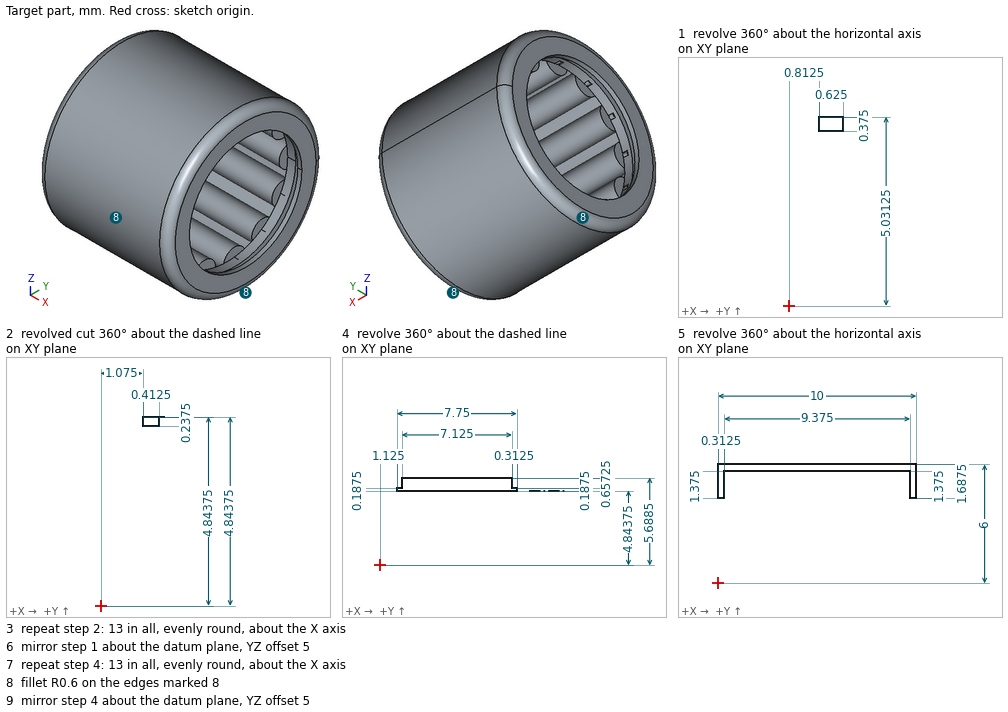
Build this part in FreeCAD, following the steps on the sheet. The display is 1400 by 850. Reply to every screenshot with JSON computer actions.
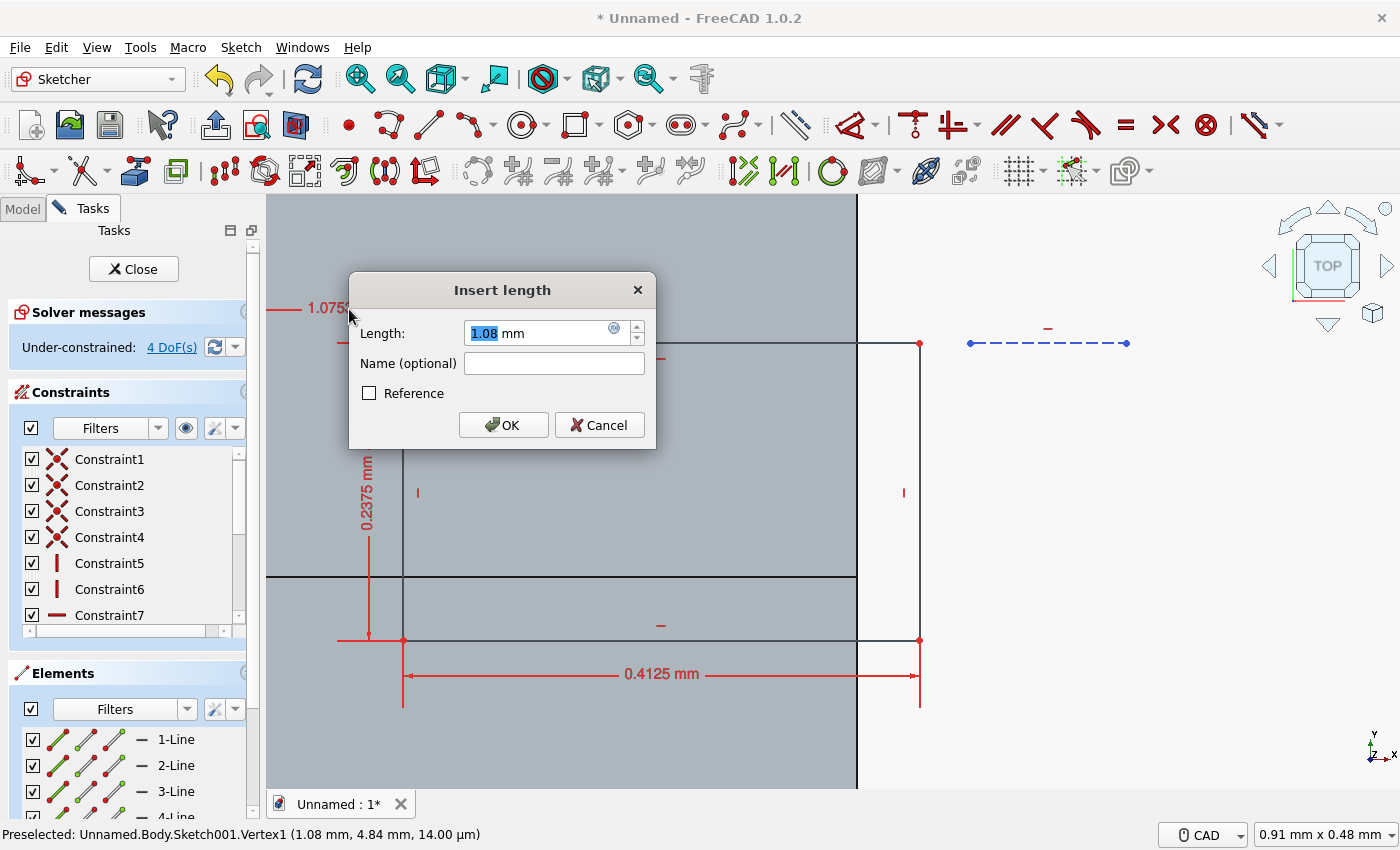
{"action": "type", "text": "1.075"}
{"action": "key", "text": "Return"}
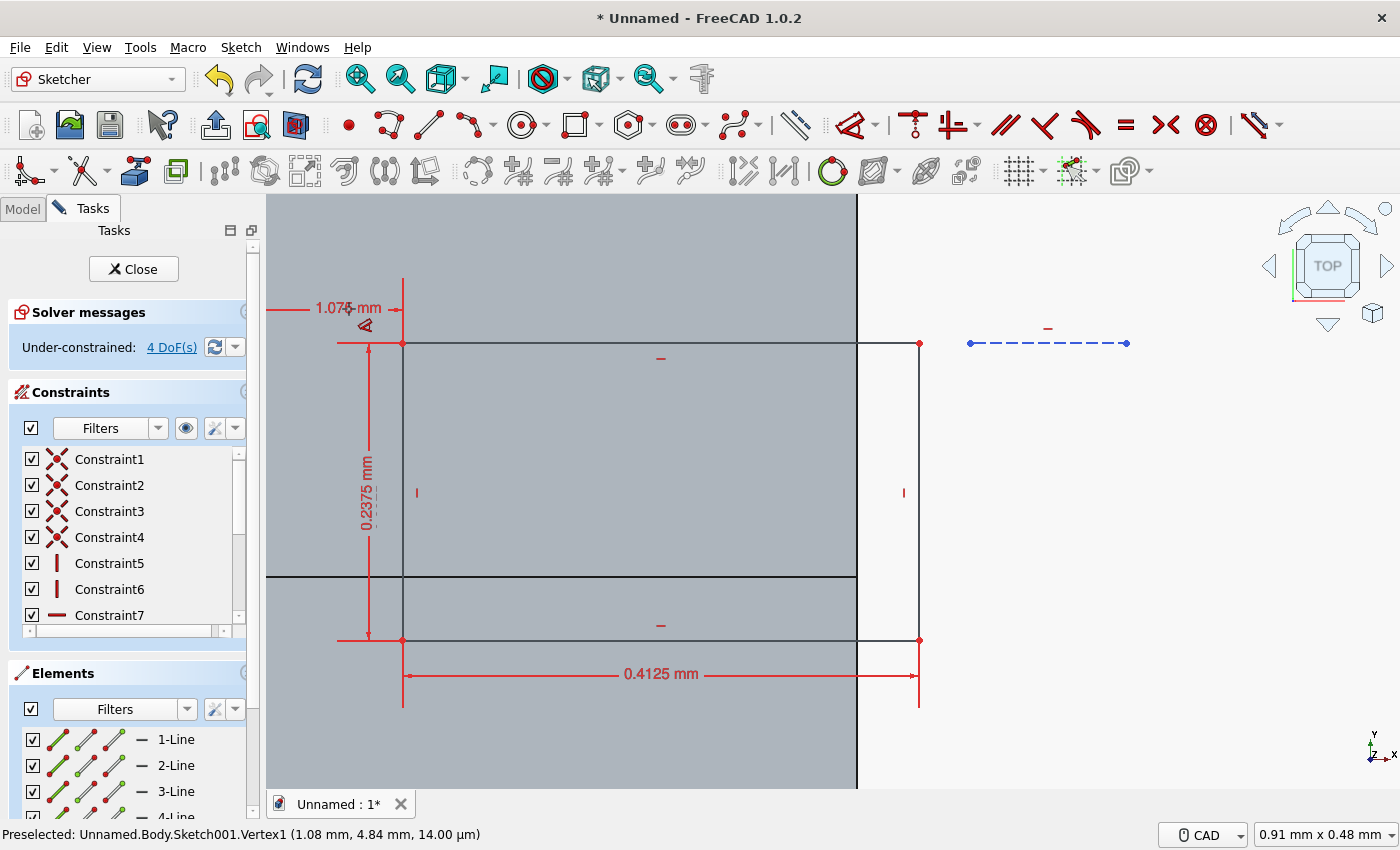
{"action": "left_click", "coordinate": [403, 343]}
{"action": "left_click", "coordinate": [437, 552]}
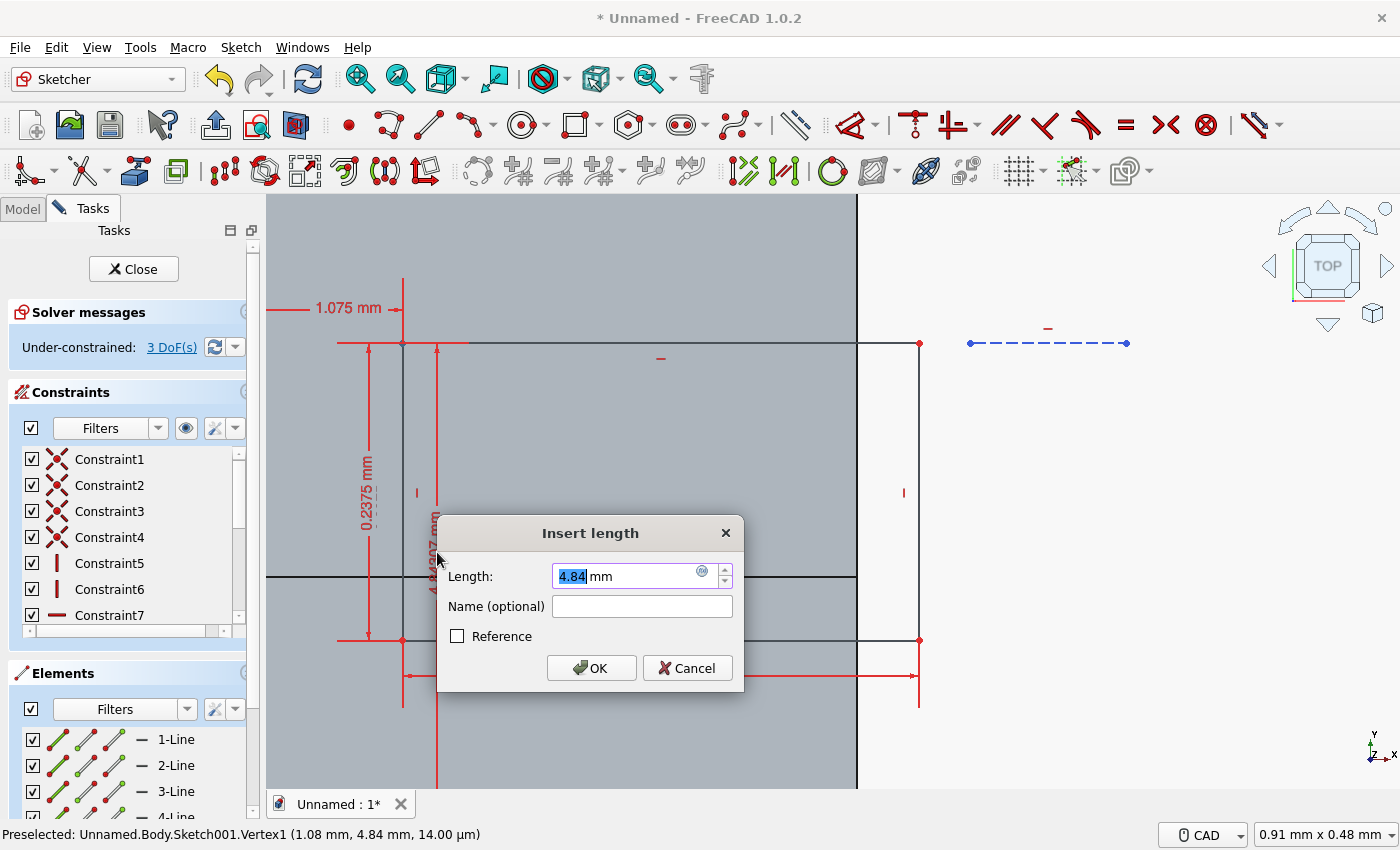
{"action": "type", "text": "4.84375"}
{"action": "key", "text": "Return"}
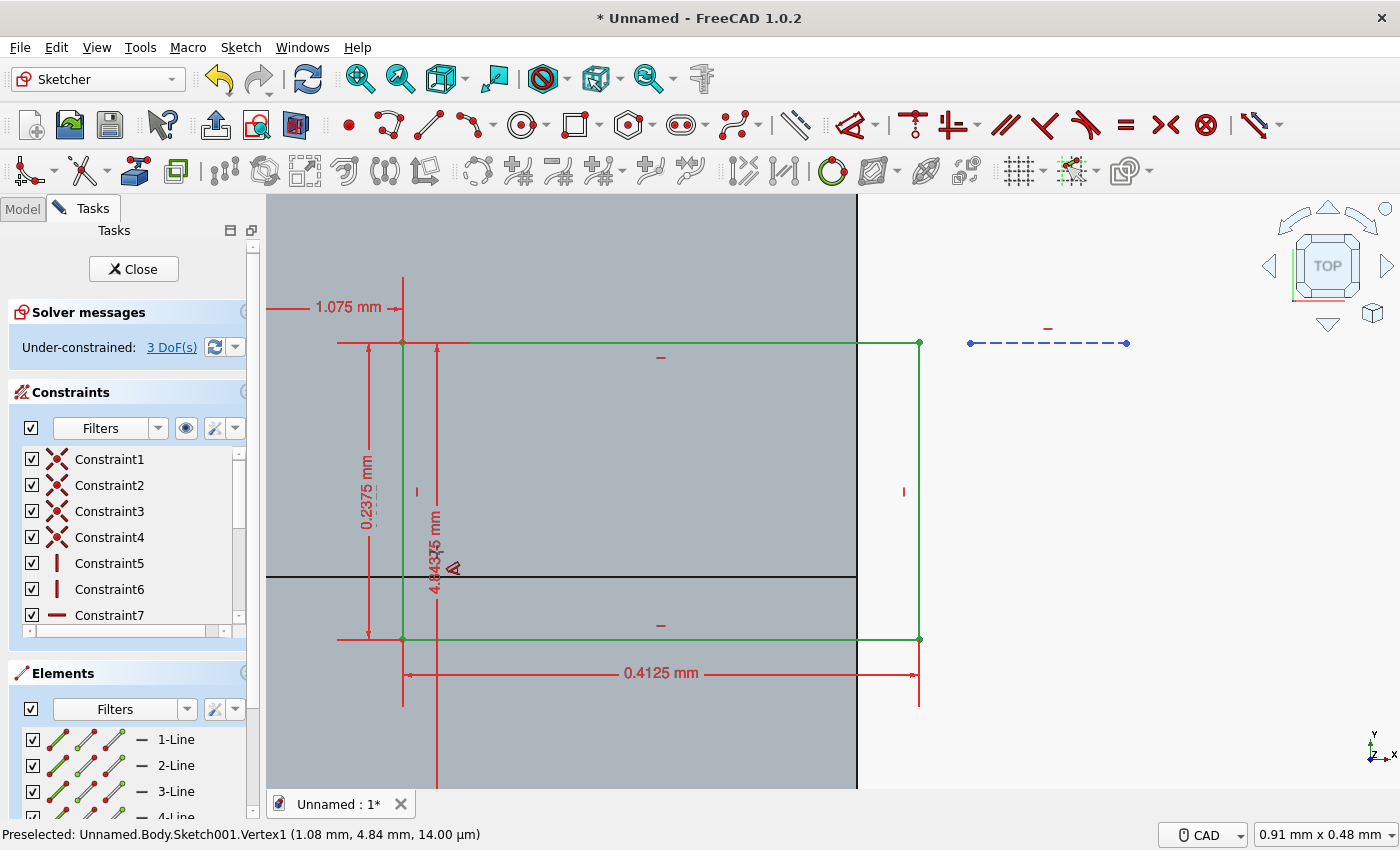
{"action": "left_click", "coordinate": [971, 343]}
{"action": "left_click", "coordinate": [1005, 552]}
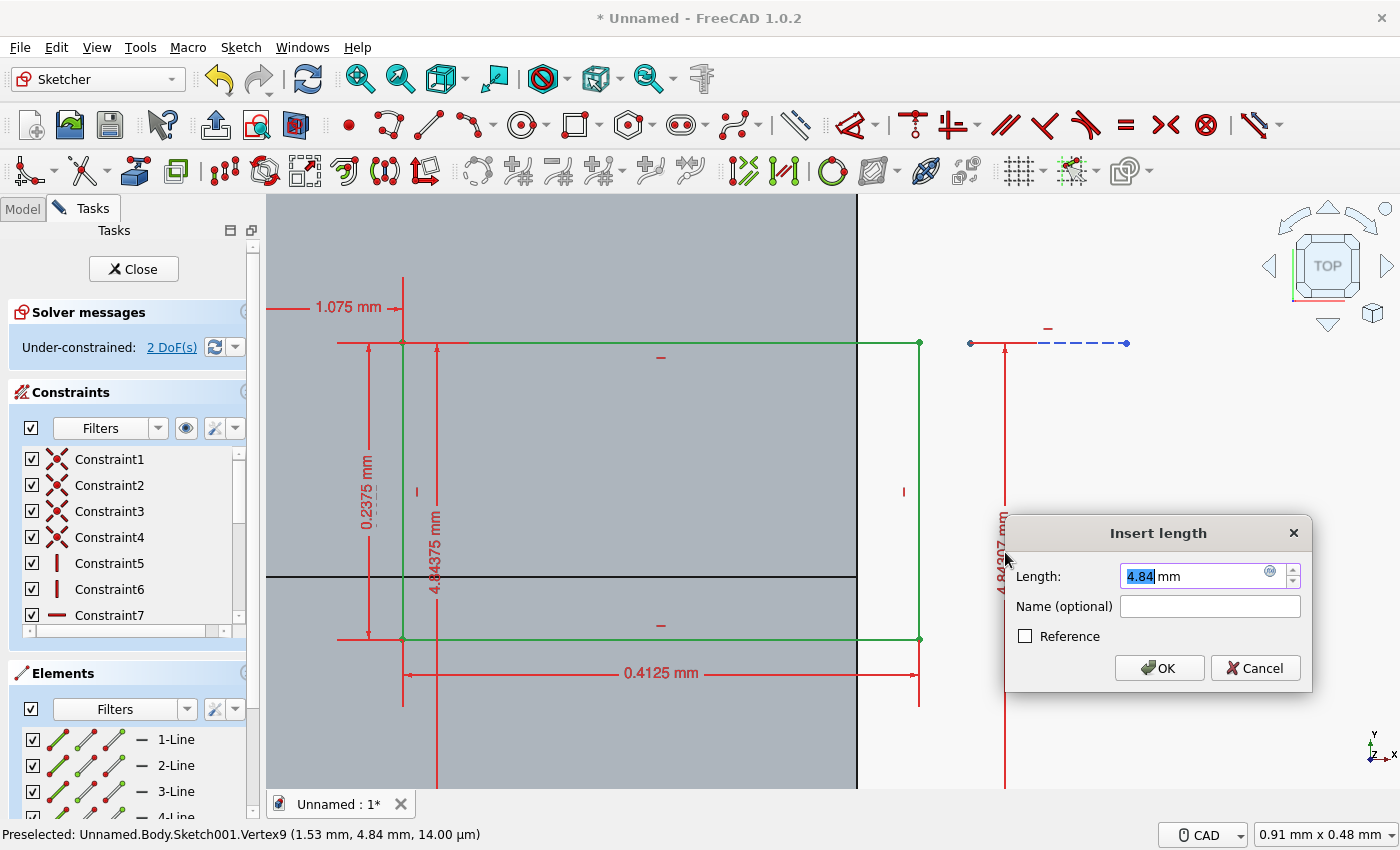
{"action": "type", "text": "4.84375"}
{"action": "key", "text": "Return"}
{"action": "key", "text": "Escape"}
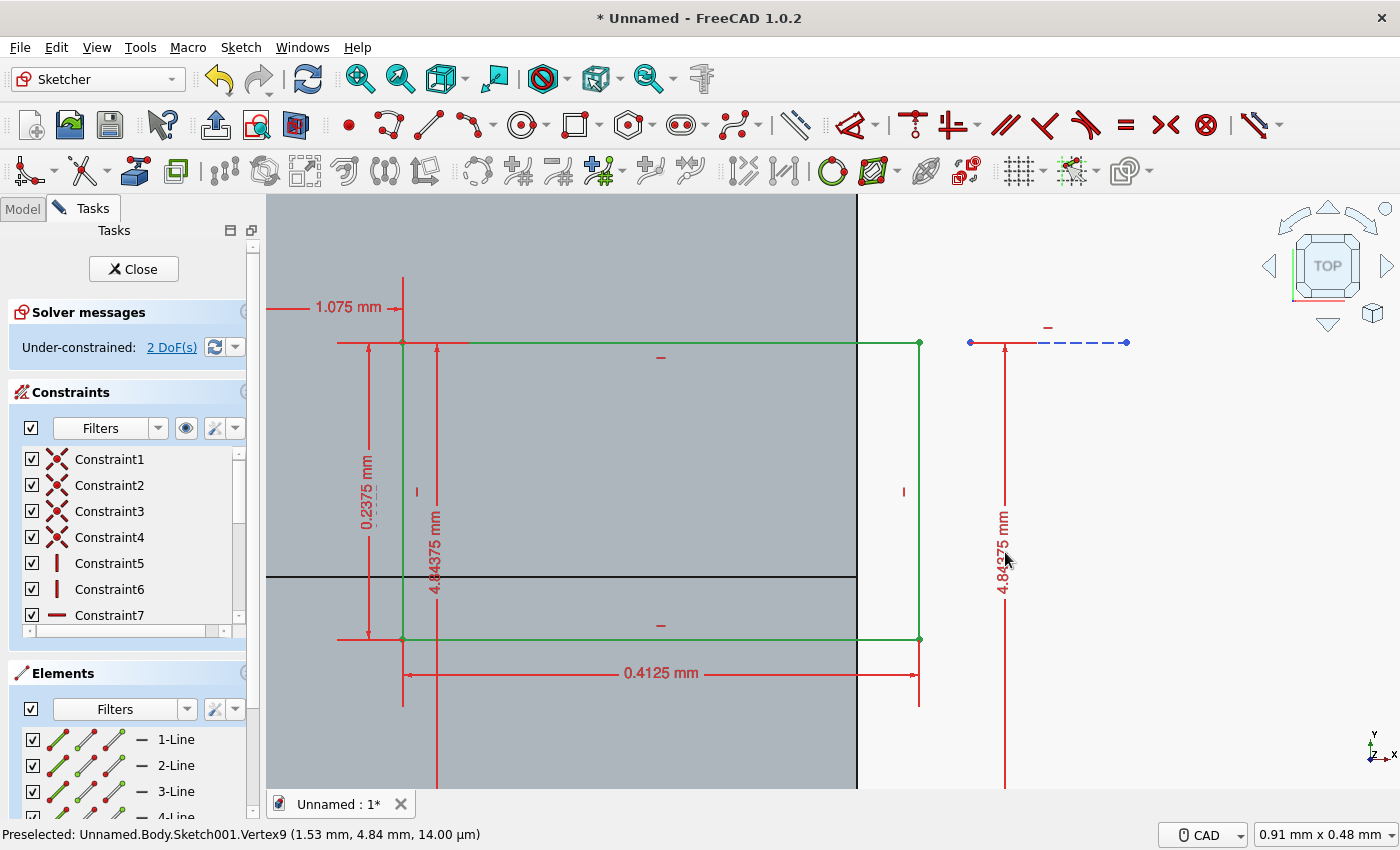
{"action": "left_click", "coordinate": [134, 269]}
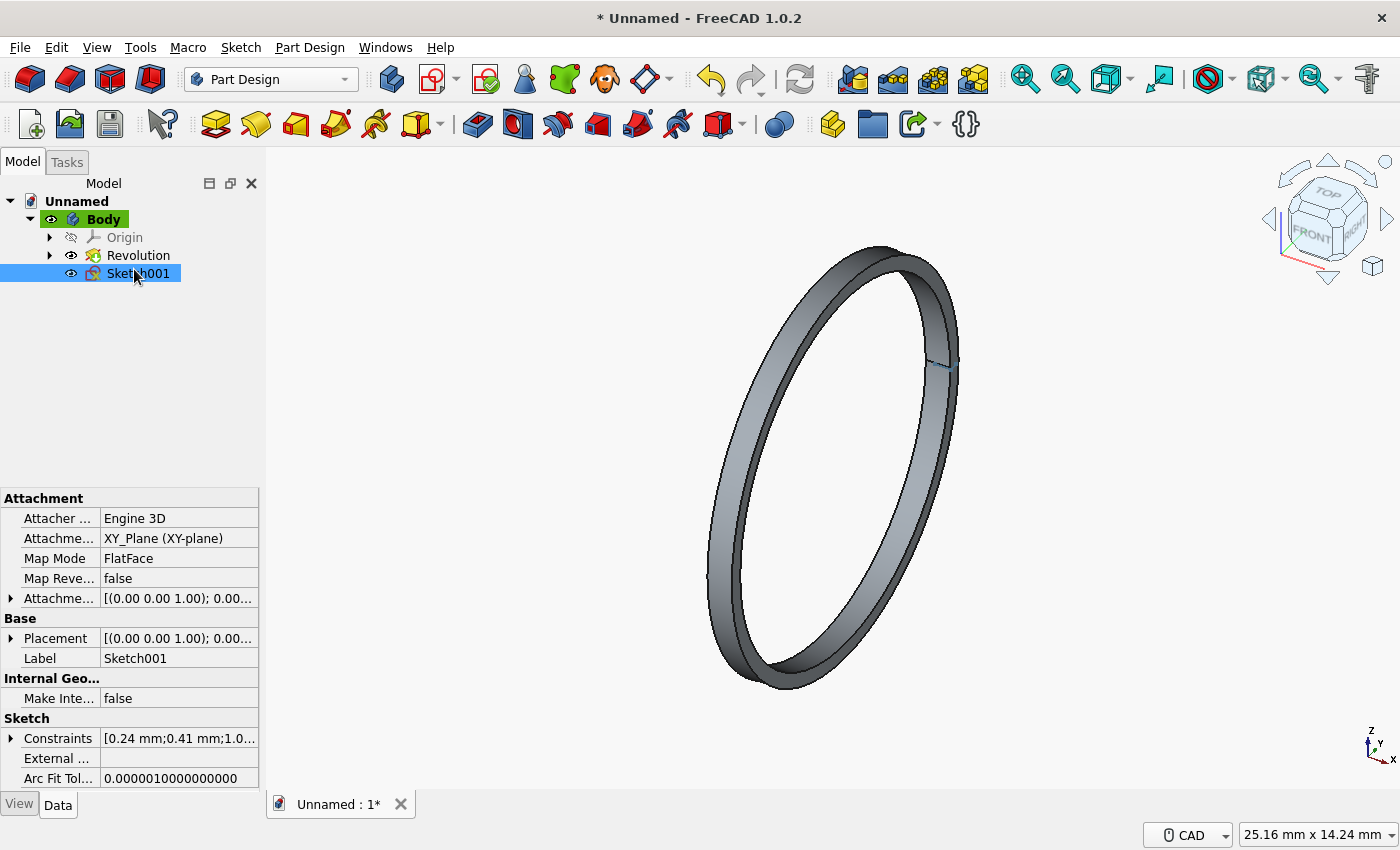
{"action": "left_click", "coordinate": [558, 124]}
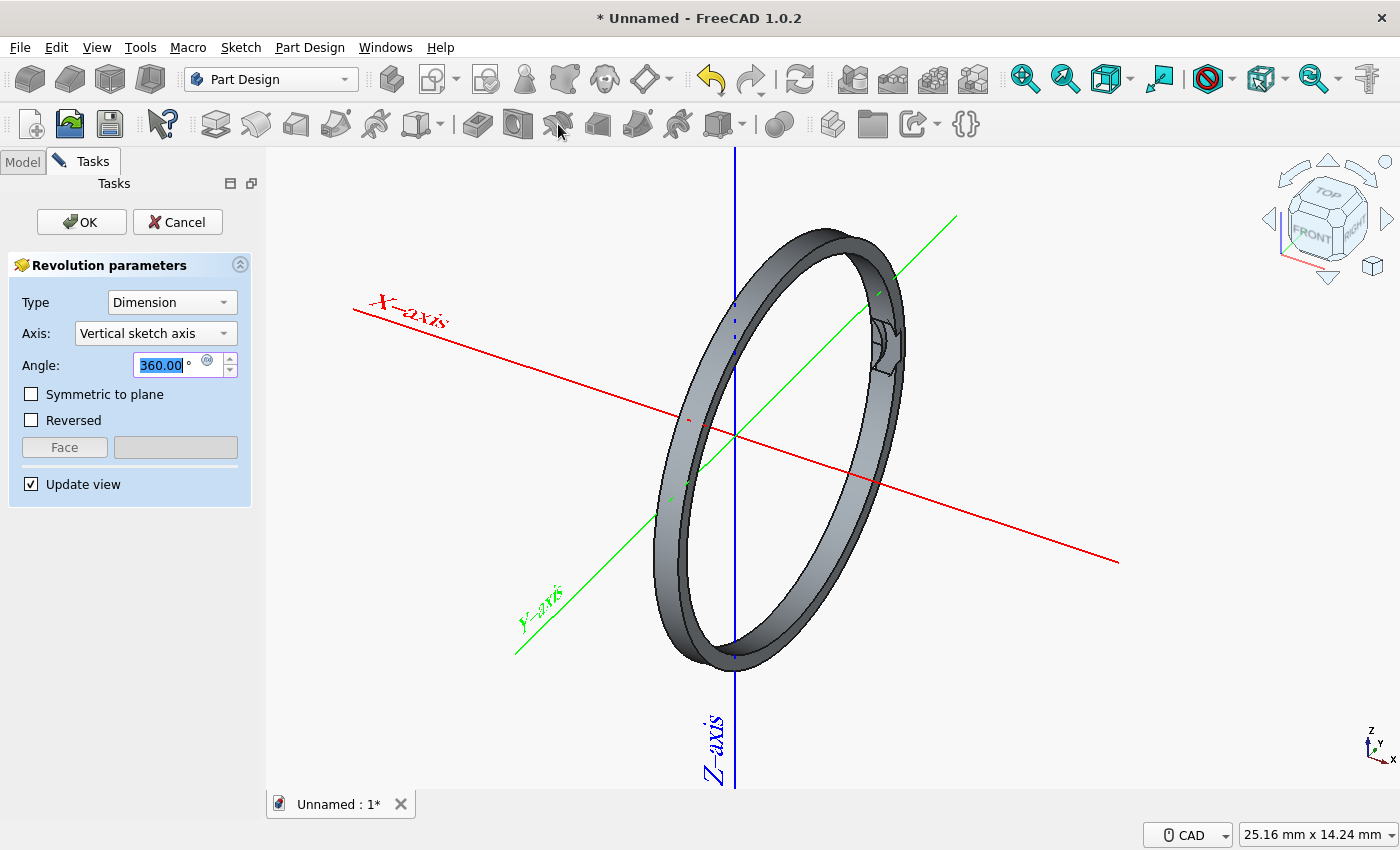
{"action": "left_click", "coordinate": [156, 334]}